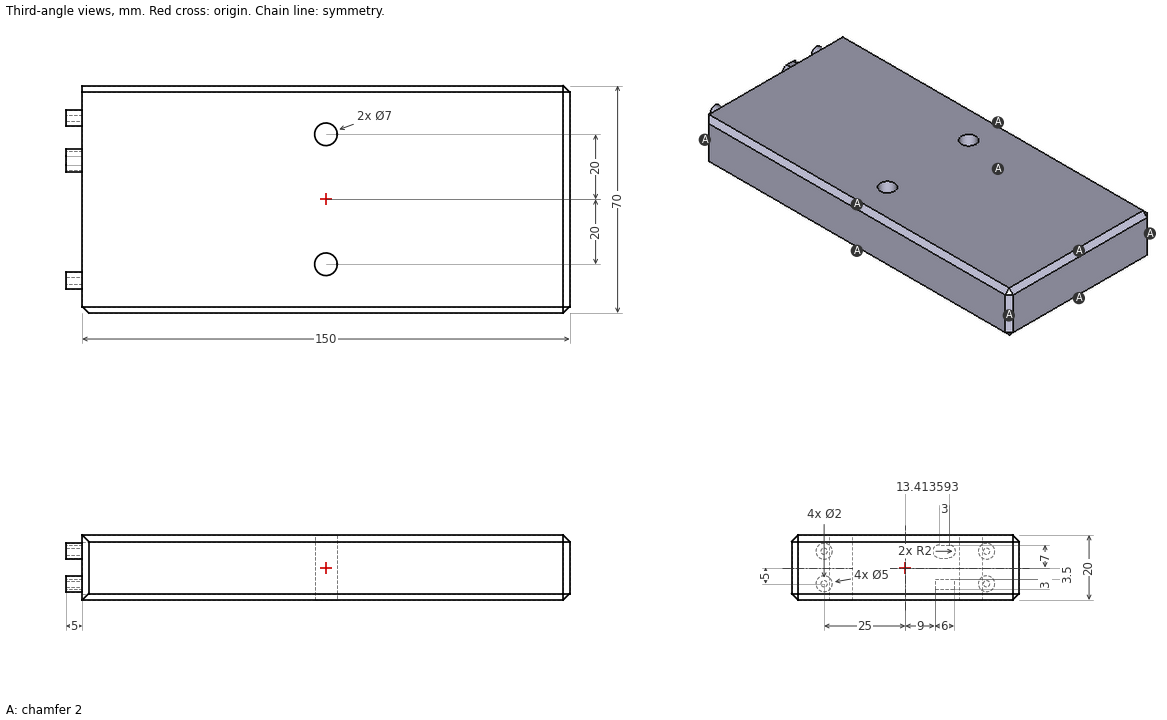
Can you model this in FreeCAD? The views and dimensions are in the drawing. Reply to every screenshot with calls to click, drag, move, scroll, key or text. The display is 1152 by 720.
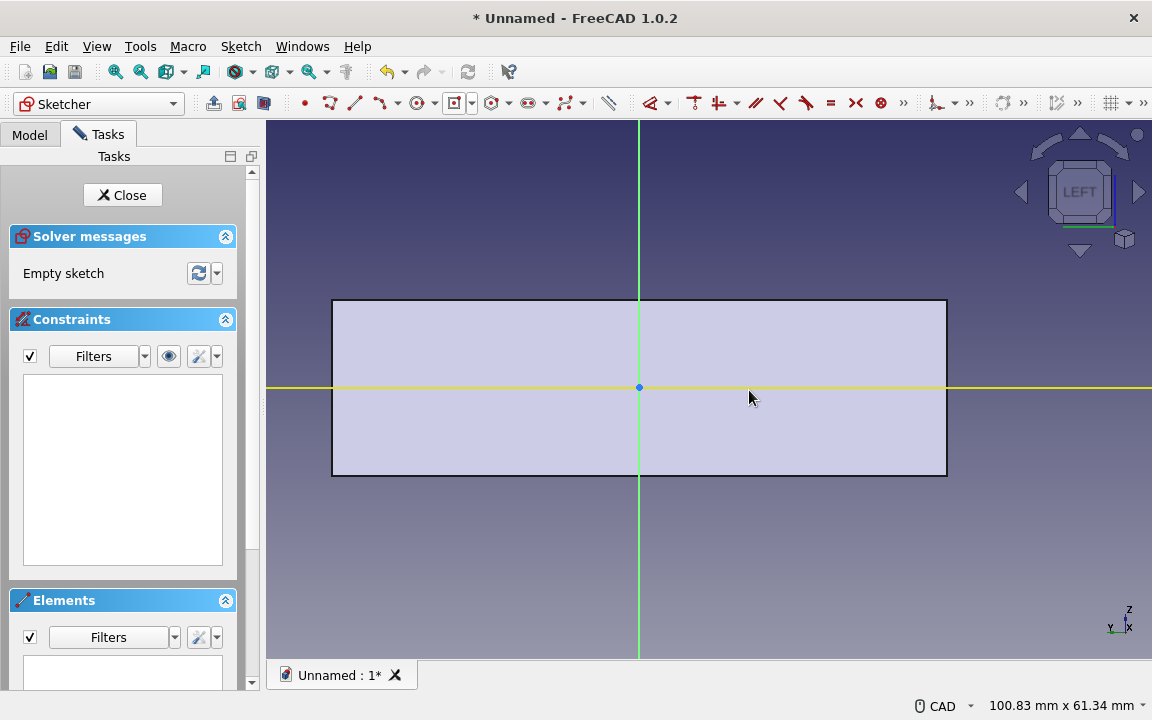
click(528, 104)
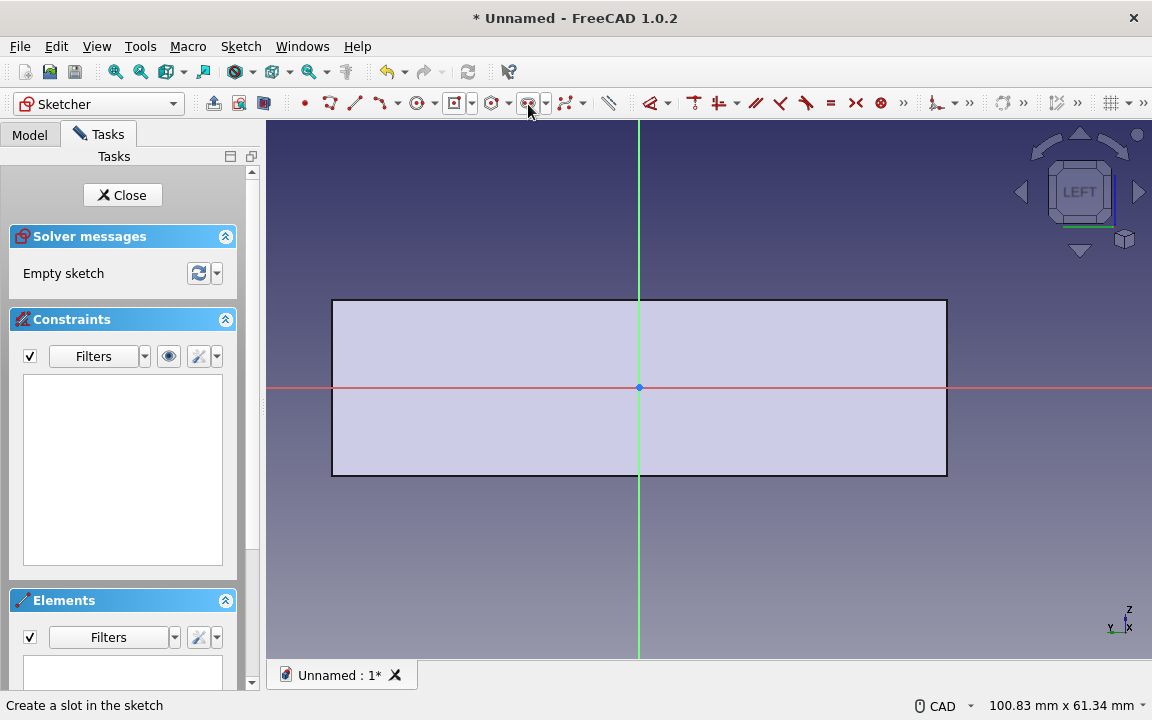
scroll(521, 344, up, 2)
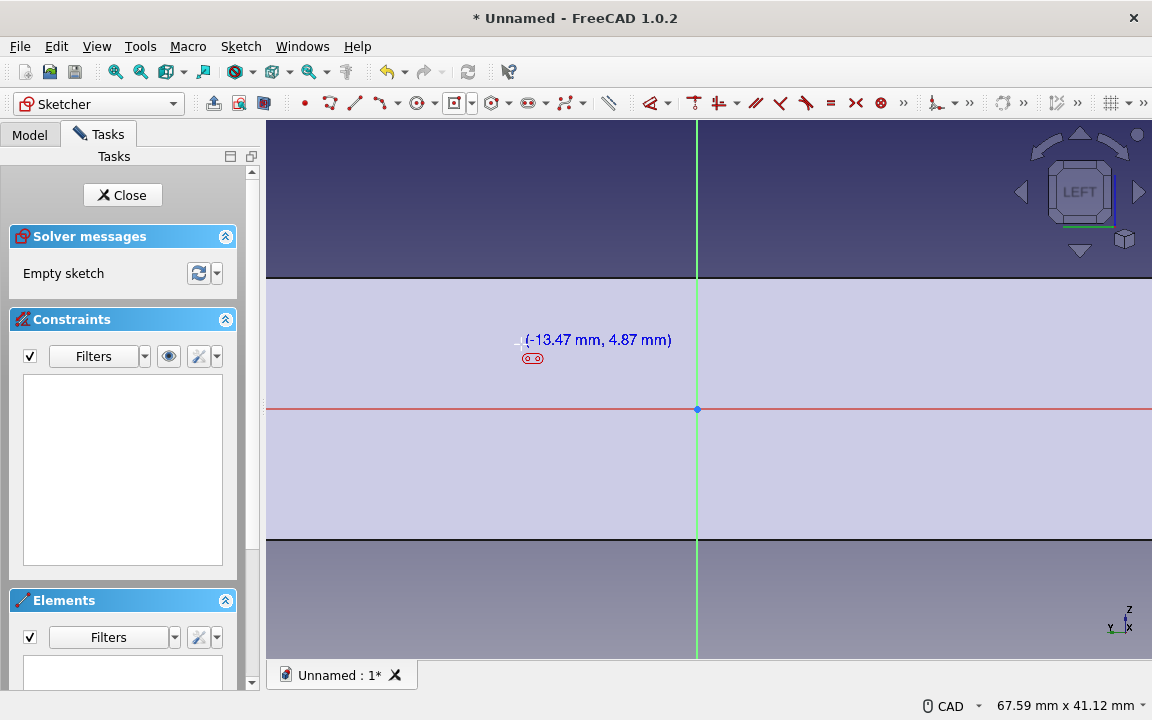
click(522, 344)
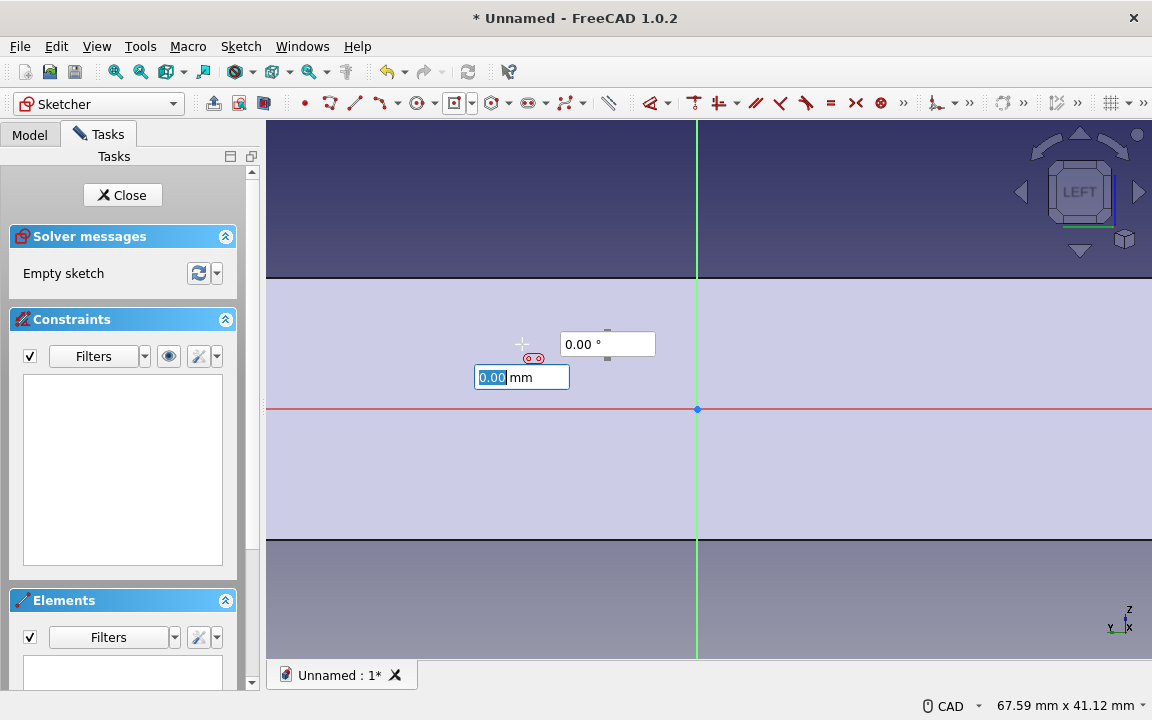
click(561, 344)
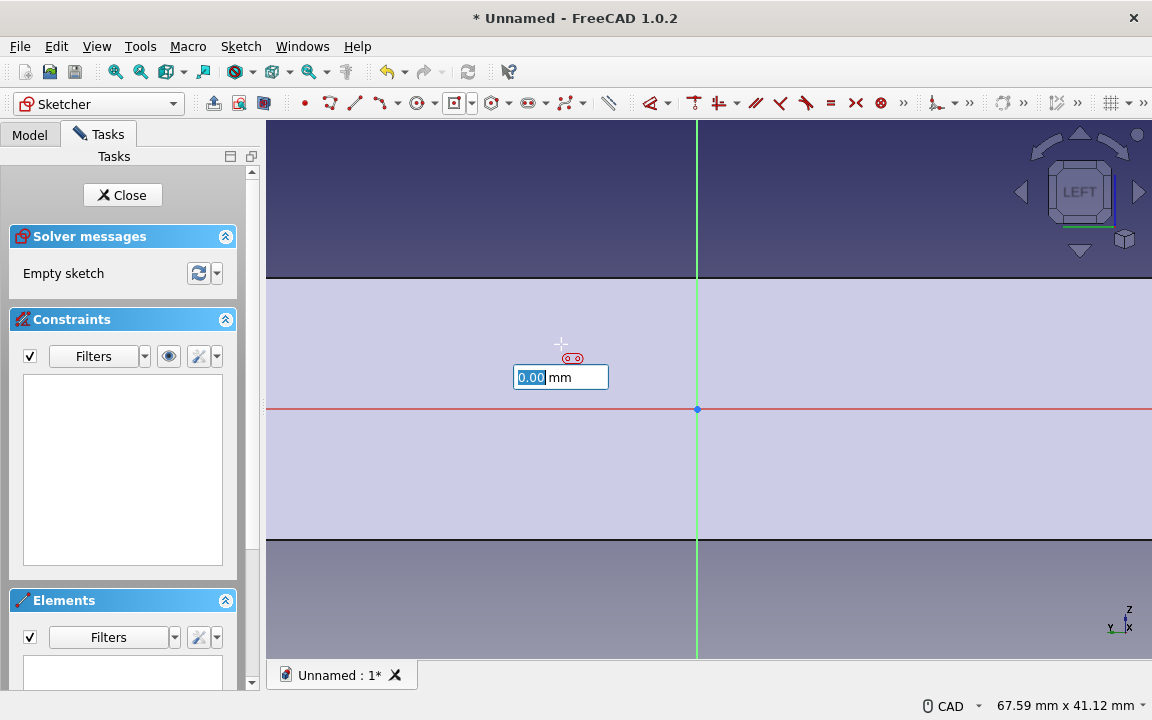
click(541, 317)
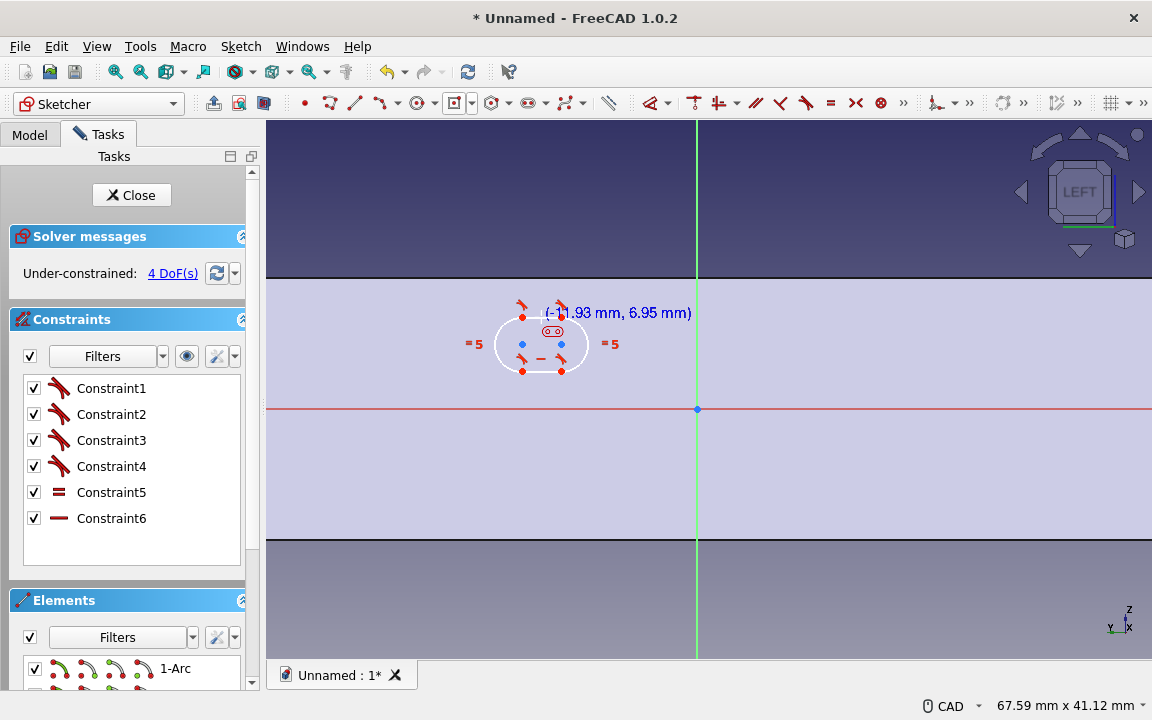
key(g)
key(r)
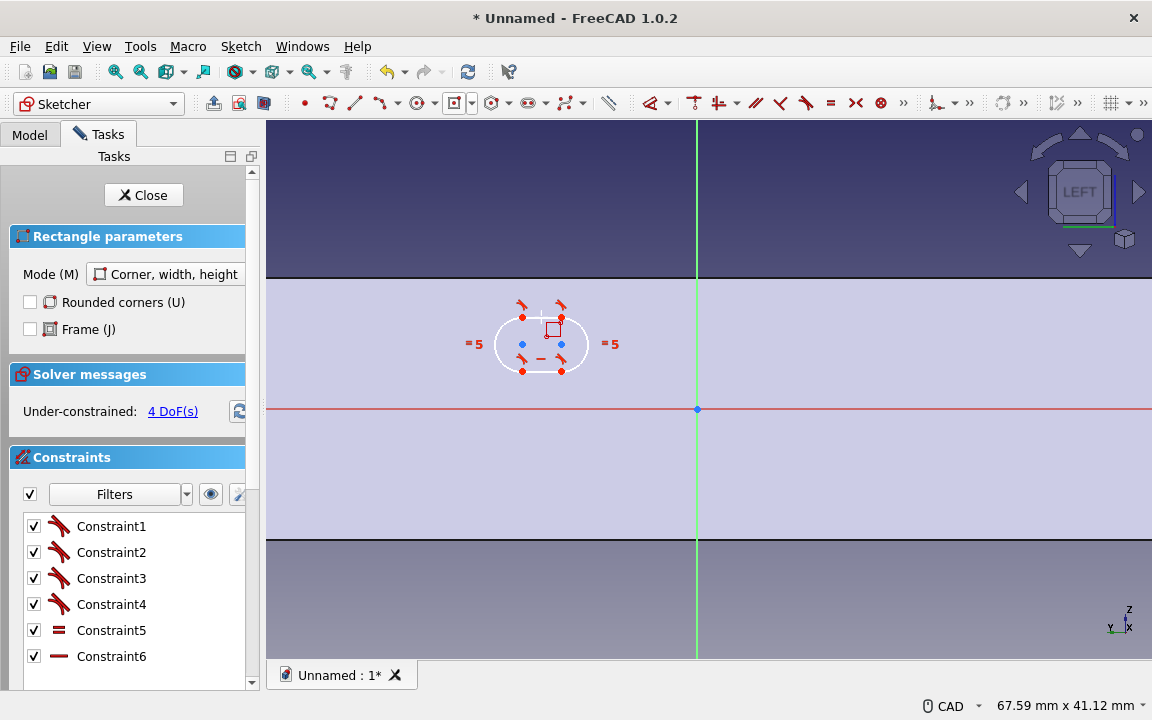
click(501, 455)
click(579, 494)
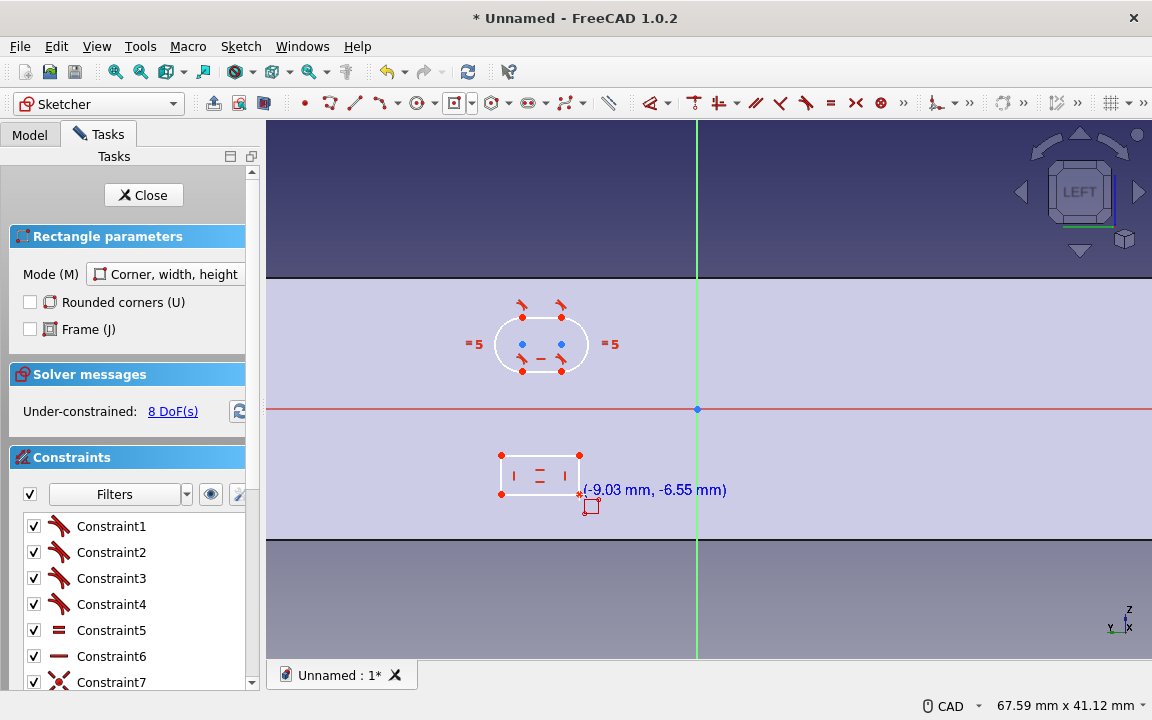
click(416, 104)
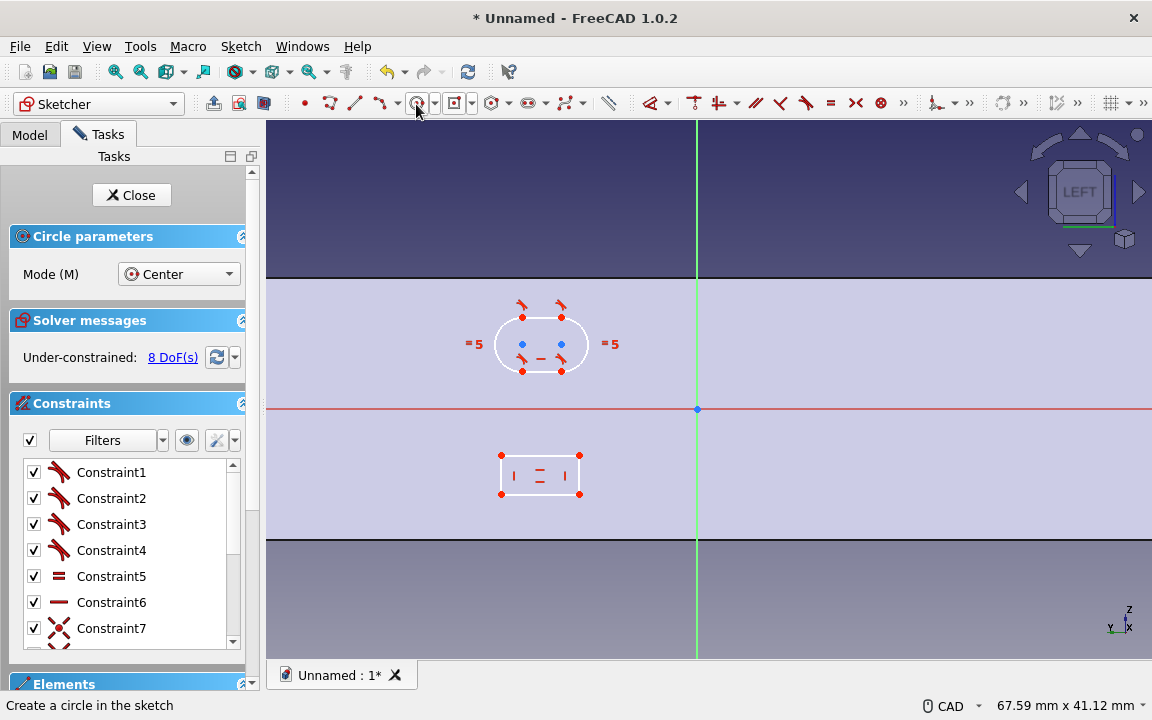
scroll(525, 350, down, 2)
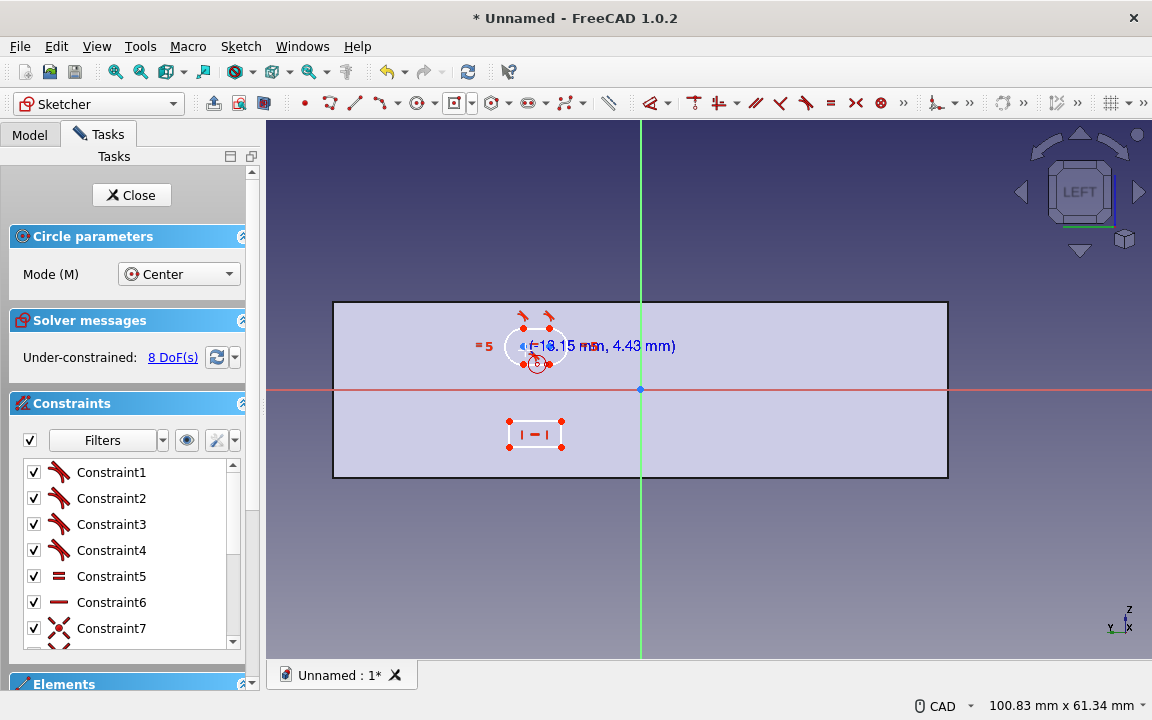
click(860, 434)
click(876, 418)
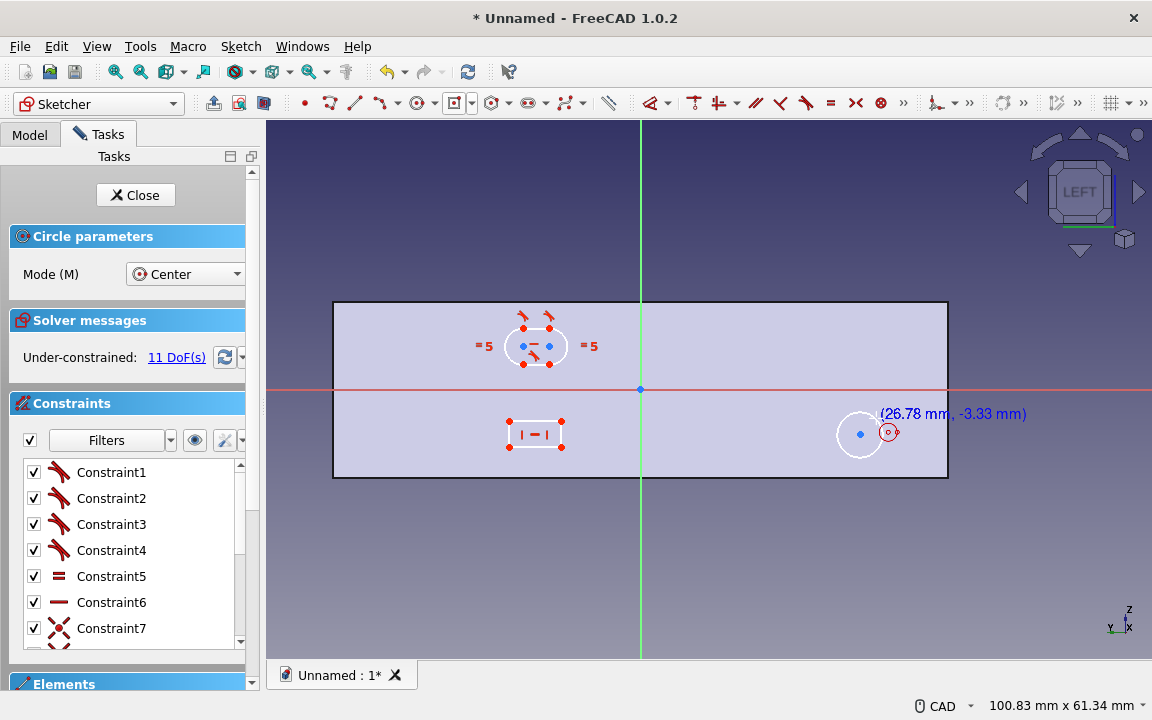
click(860, 346)
click(876, 330)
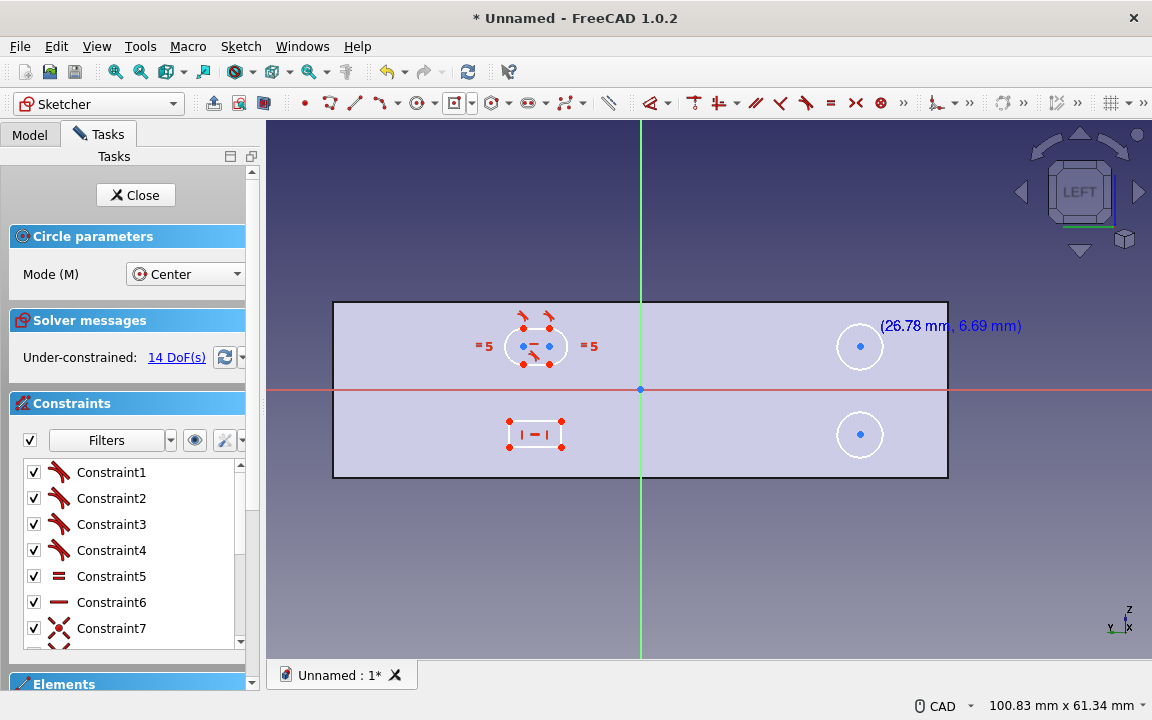
click(421, 346)
click(437, 330)